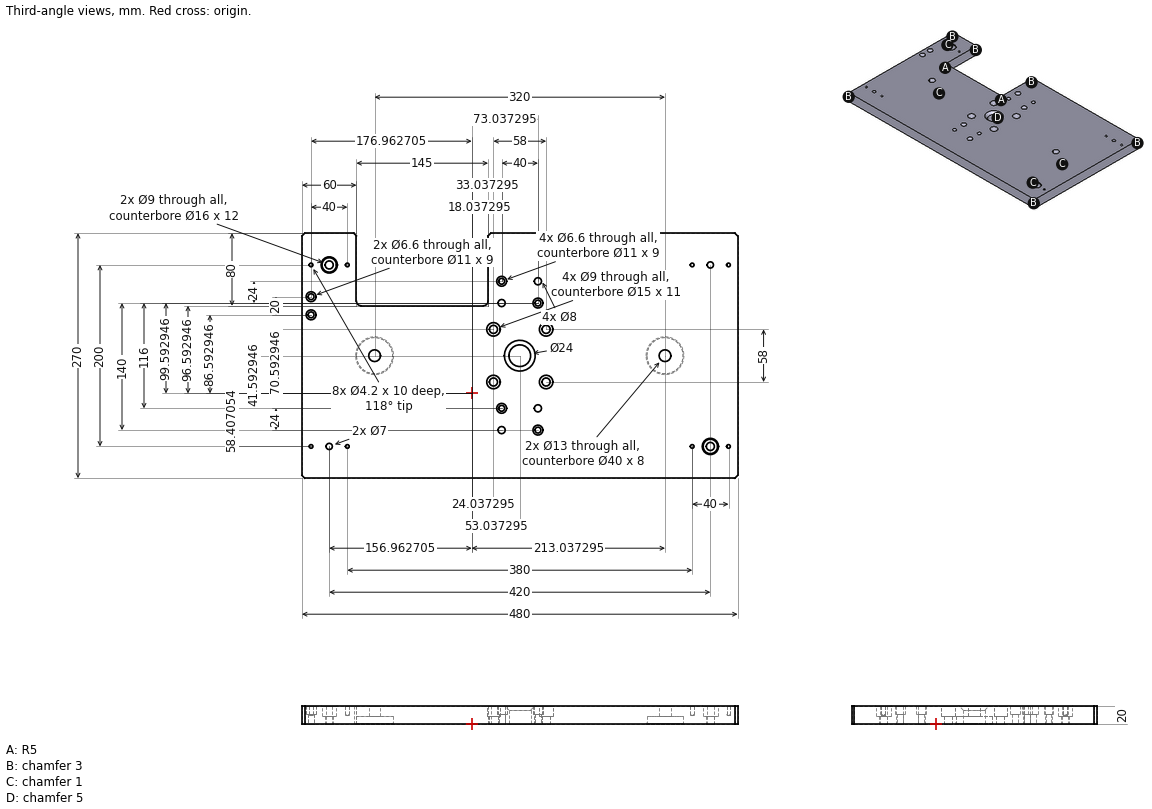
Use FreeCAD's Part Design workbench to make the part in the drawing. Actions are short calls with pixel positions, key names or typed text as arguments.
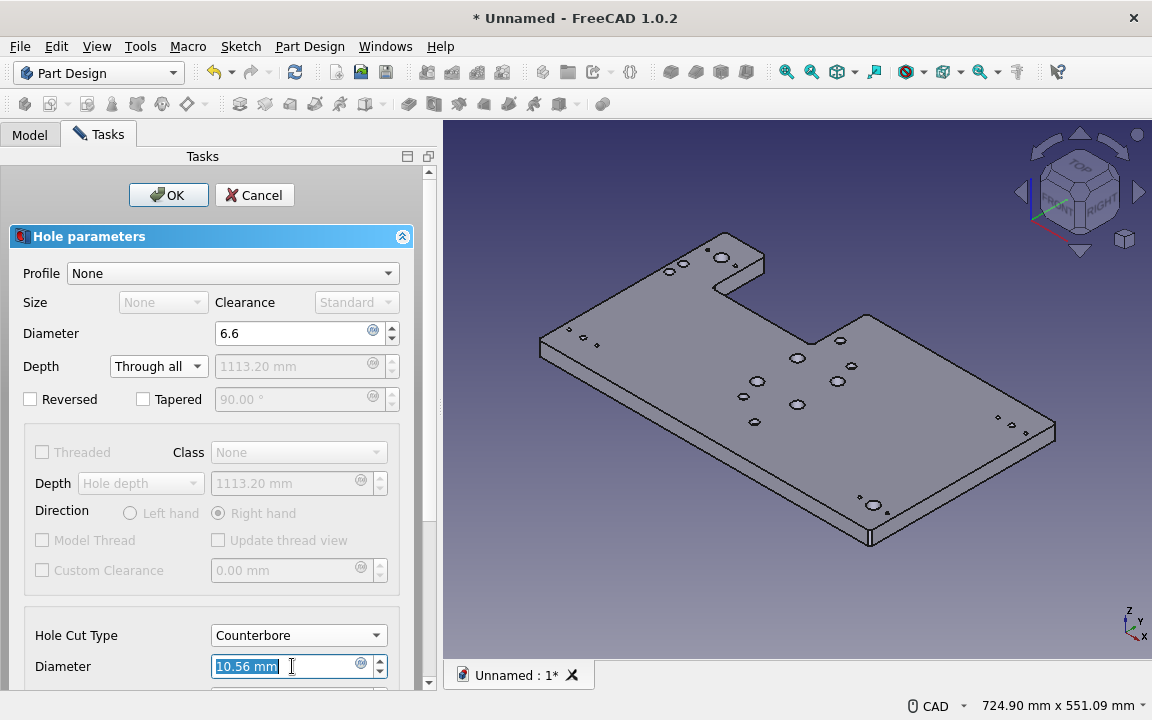
text(11)
key(Tab)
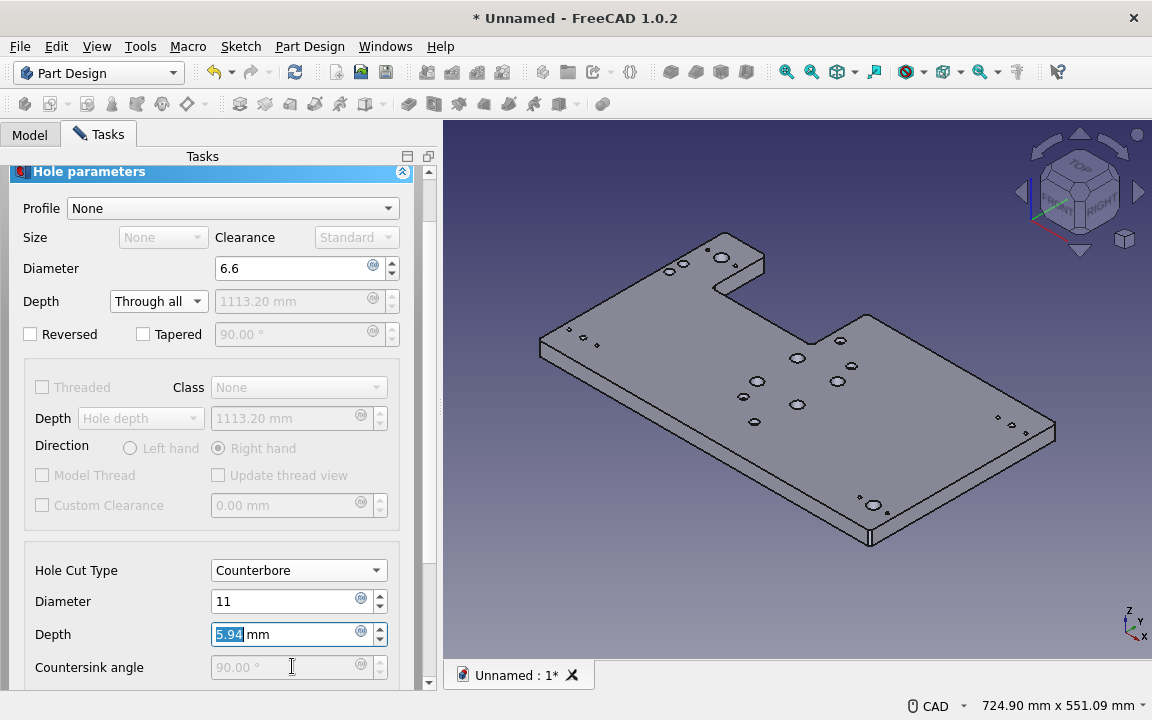
text(9)
key(Tab)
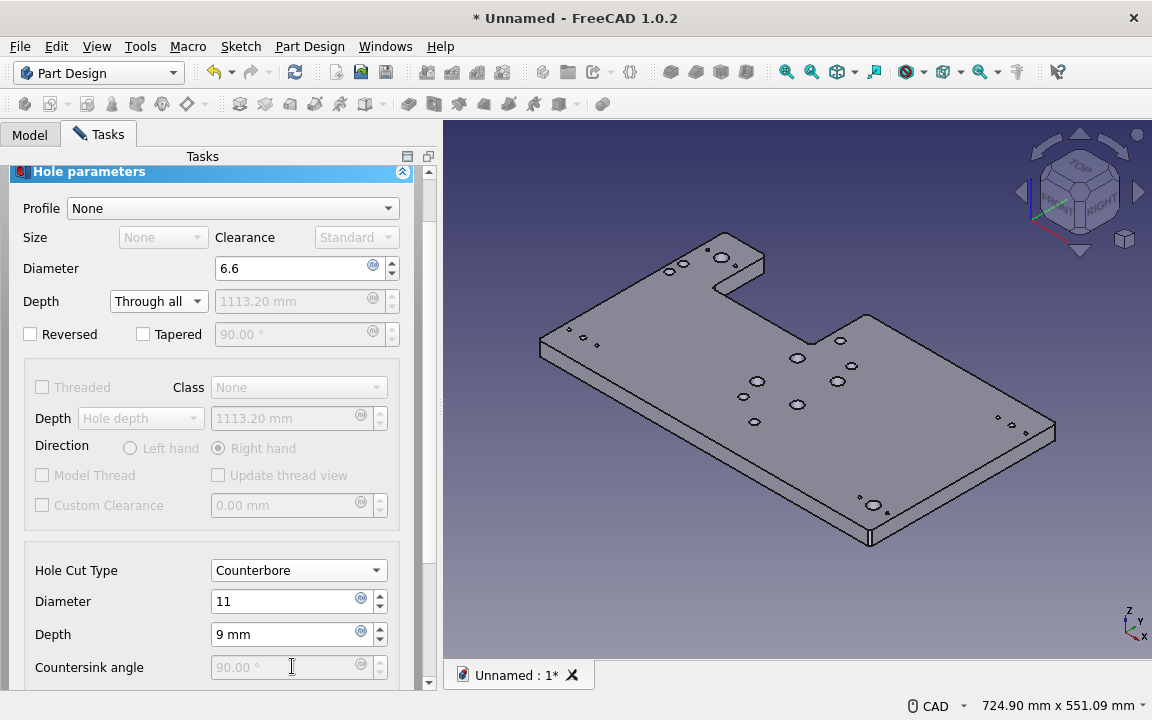
scroll(429, 428, up, 2)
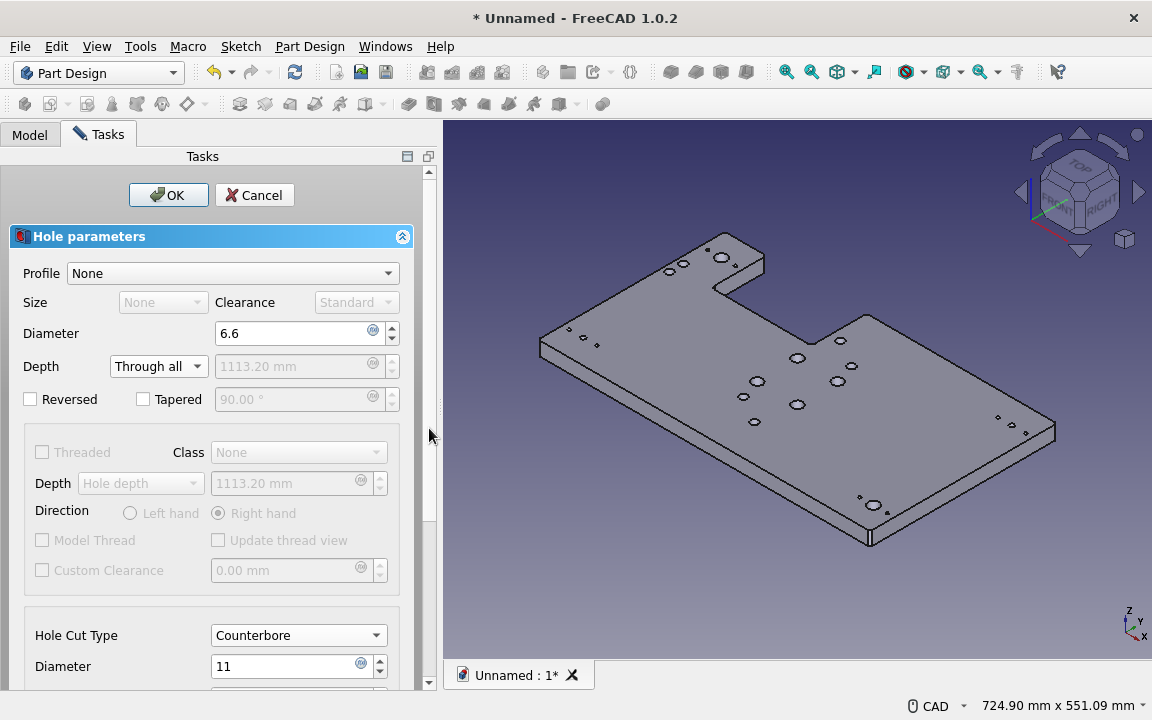
click(169, 195)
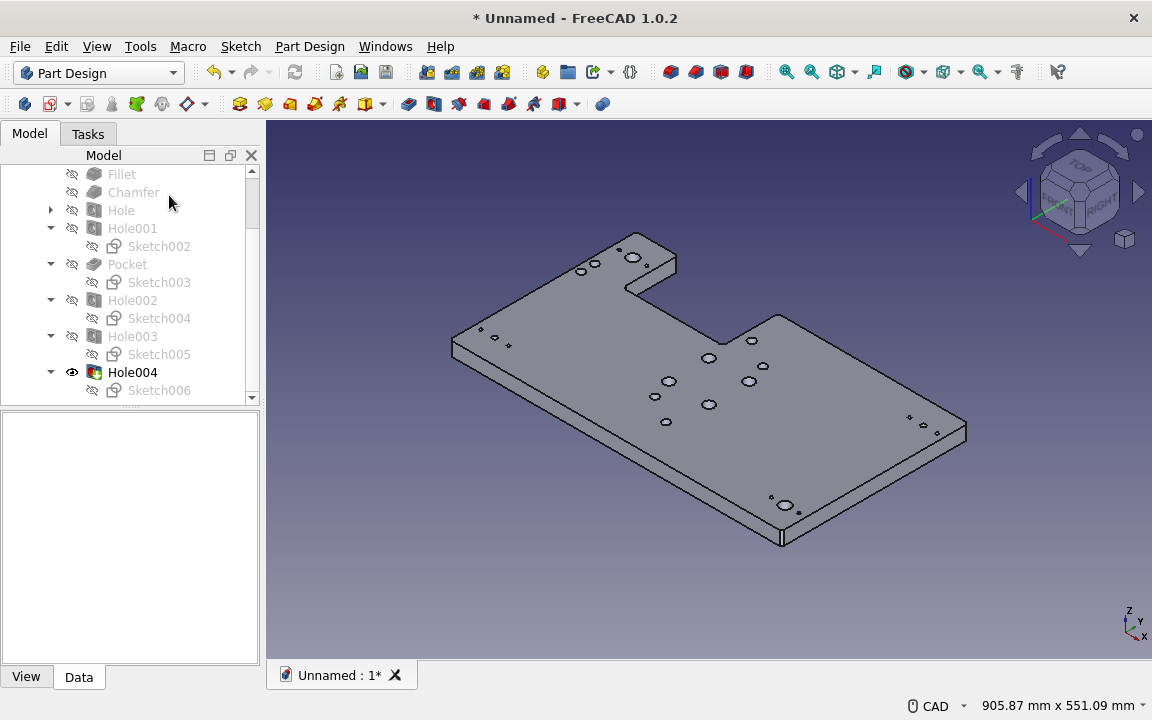
click(804, 435)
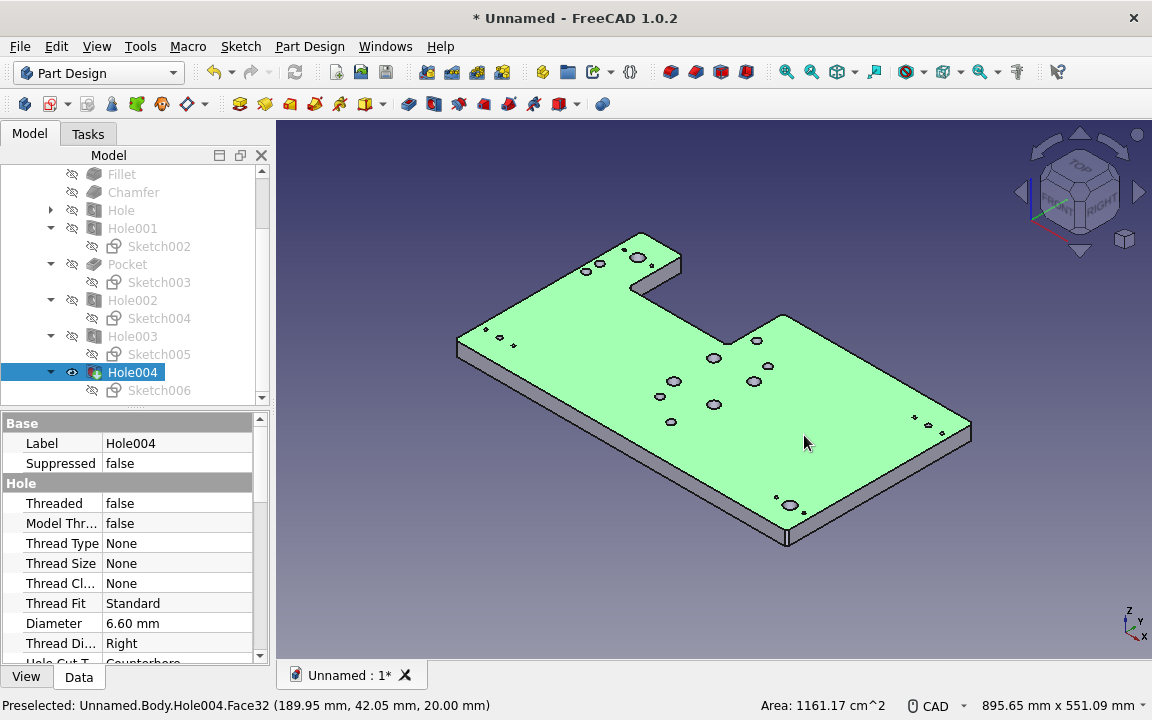
click(50, 104)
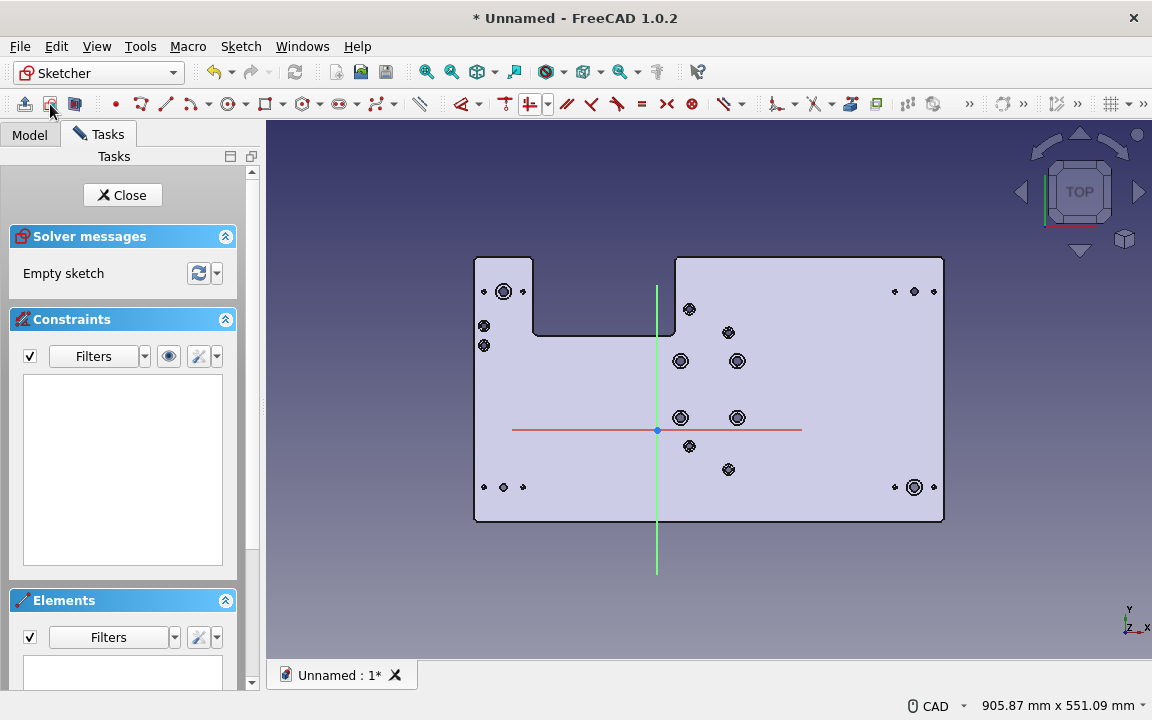
scroll(739, 390, up, 4)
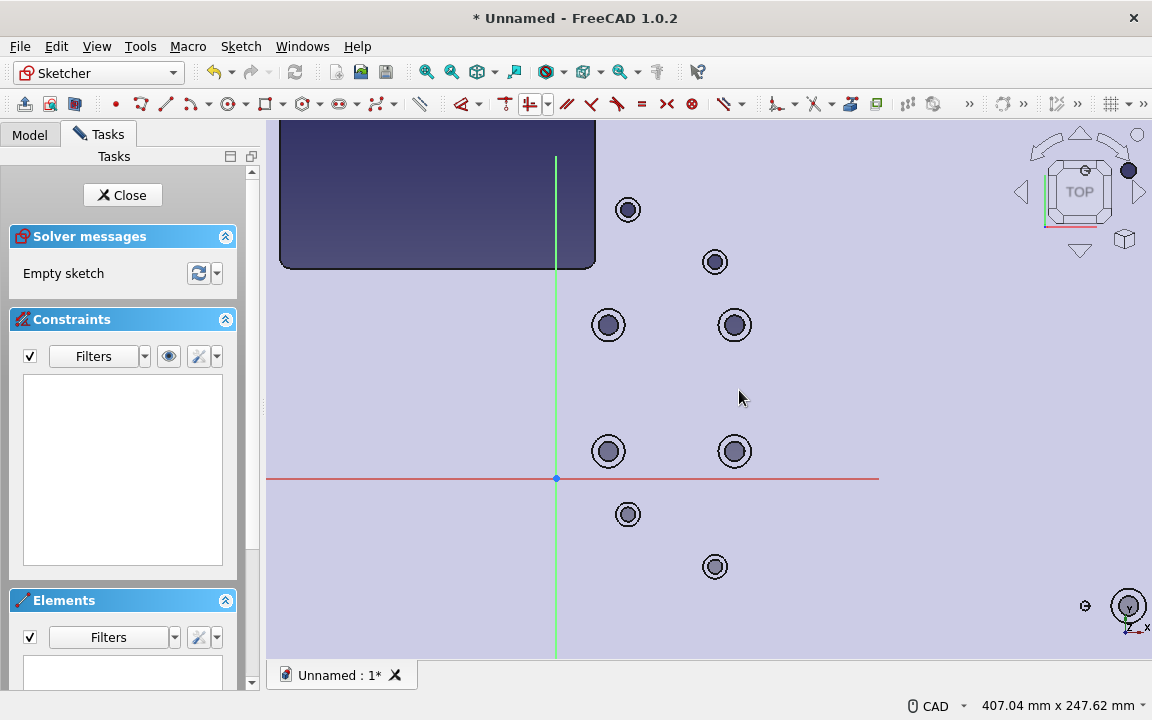
key(g)
key(c)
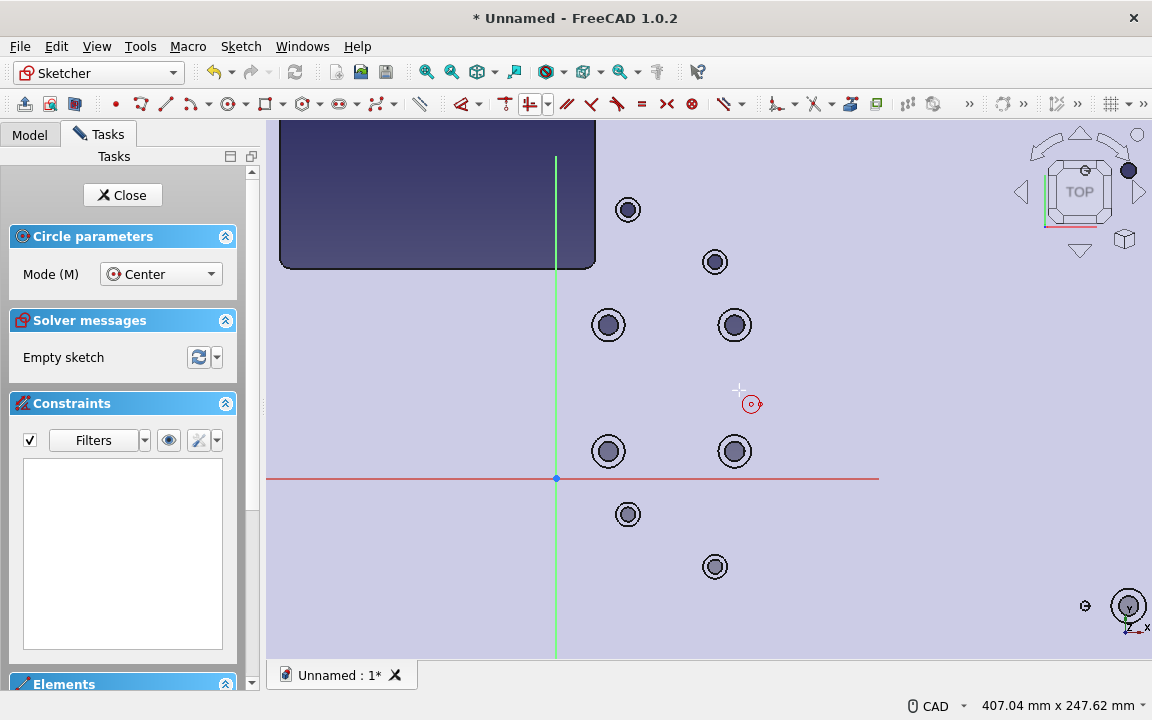
scroll(715, 210, up, 5)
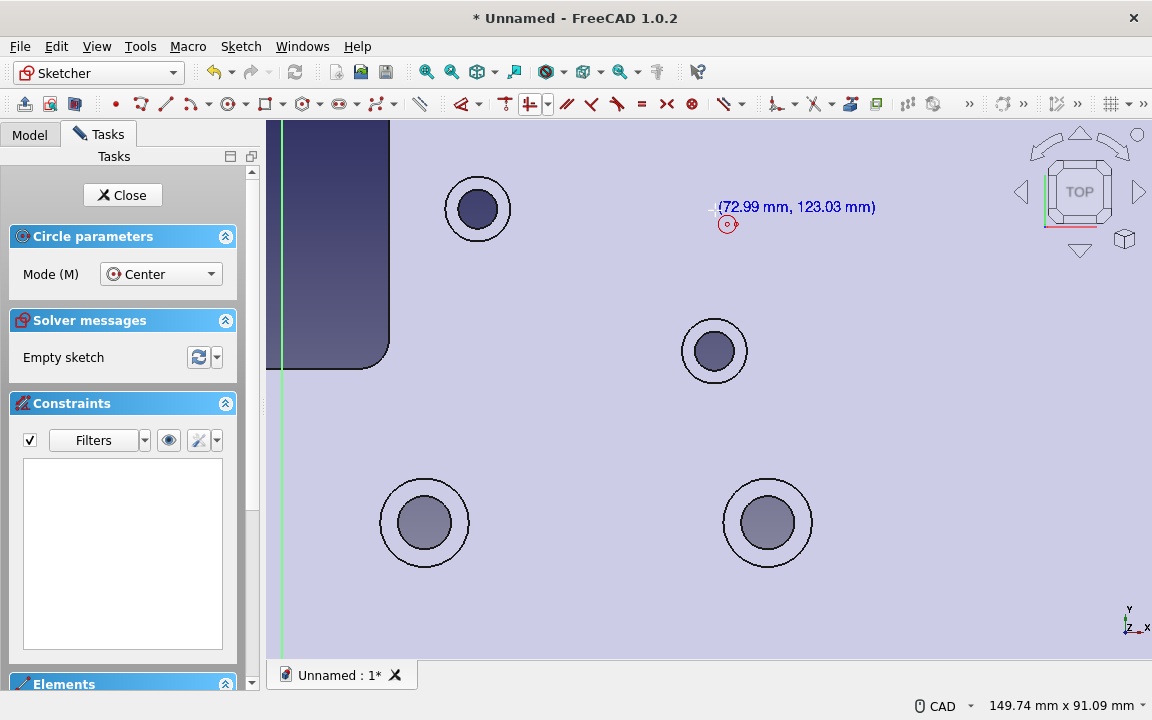
click(714, 209)
click(731, 192)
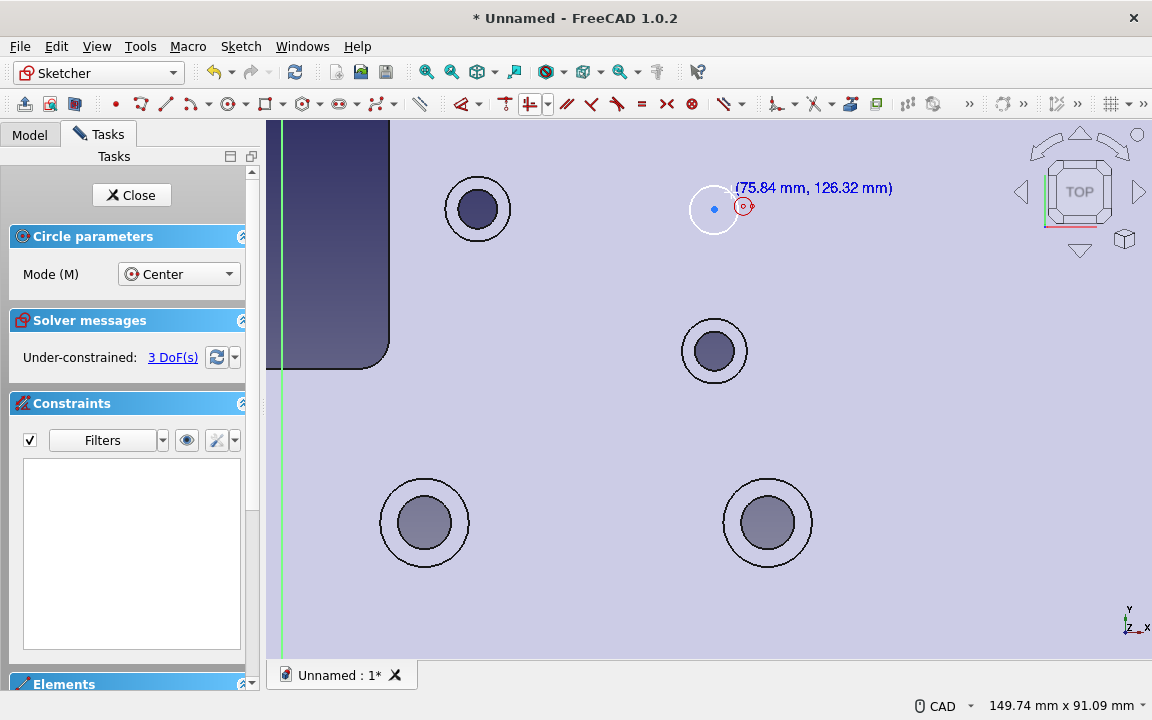
click(478, 351)
click(494, 334)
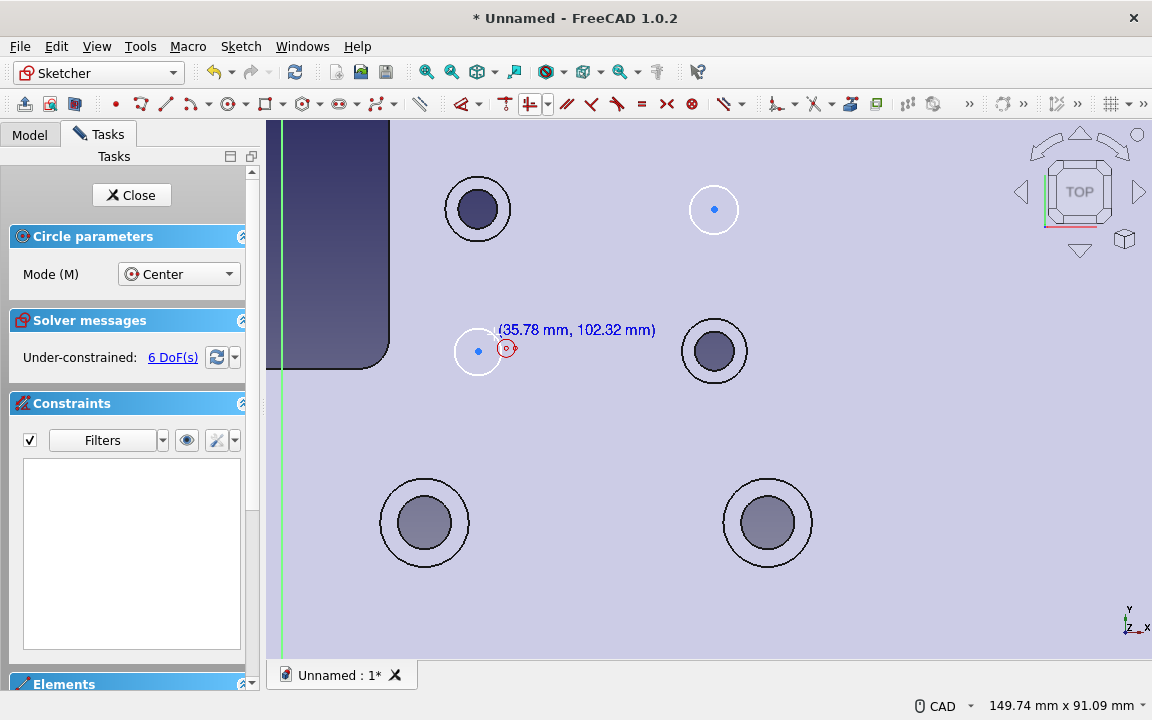
scroll(716, 212, down, 5)